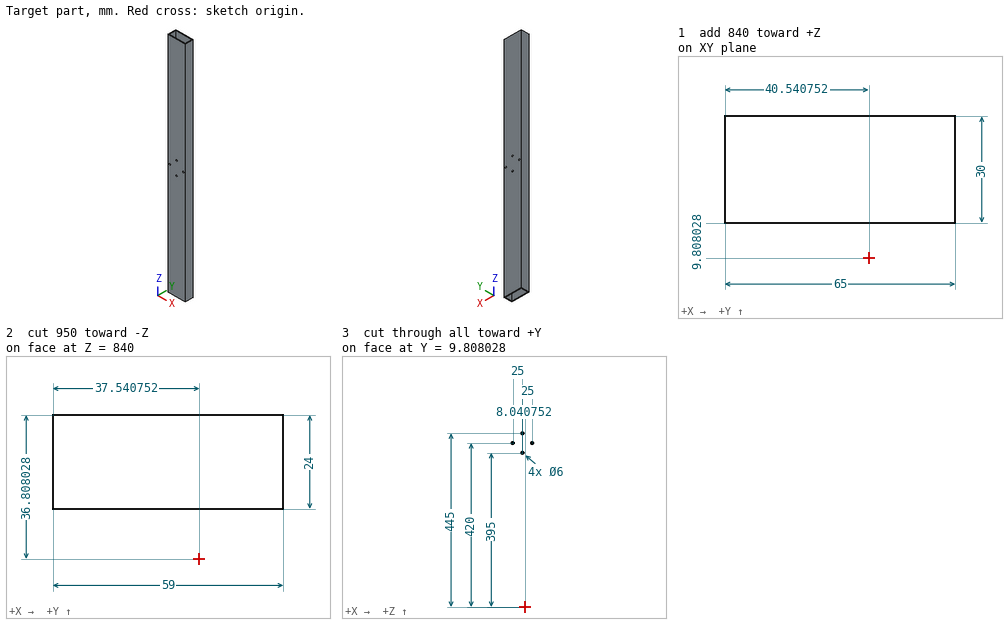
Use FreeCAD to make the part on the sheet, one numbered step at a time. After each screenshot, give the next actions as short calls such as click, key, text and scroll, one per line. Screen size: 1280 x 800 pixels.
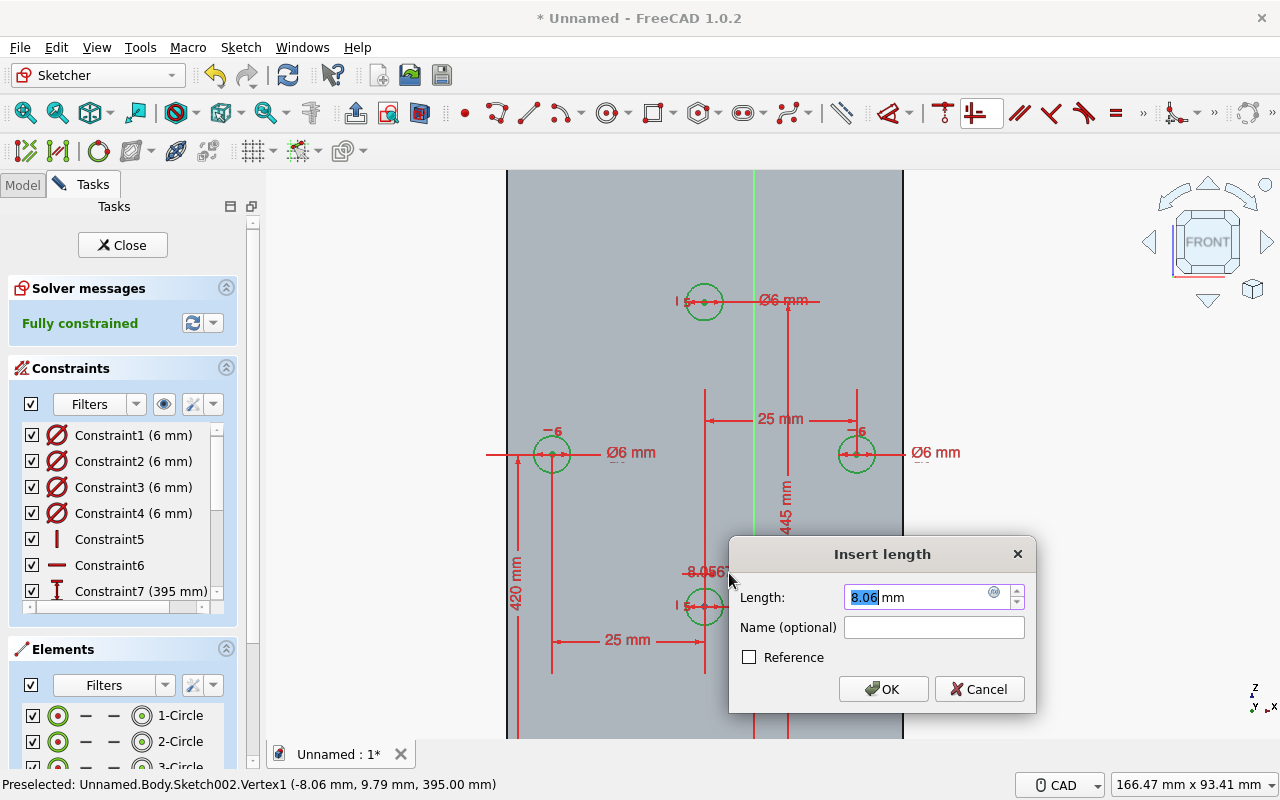
text(8.040752)
key(Return)
key(Escape)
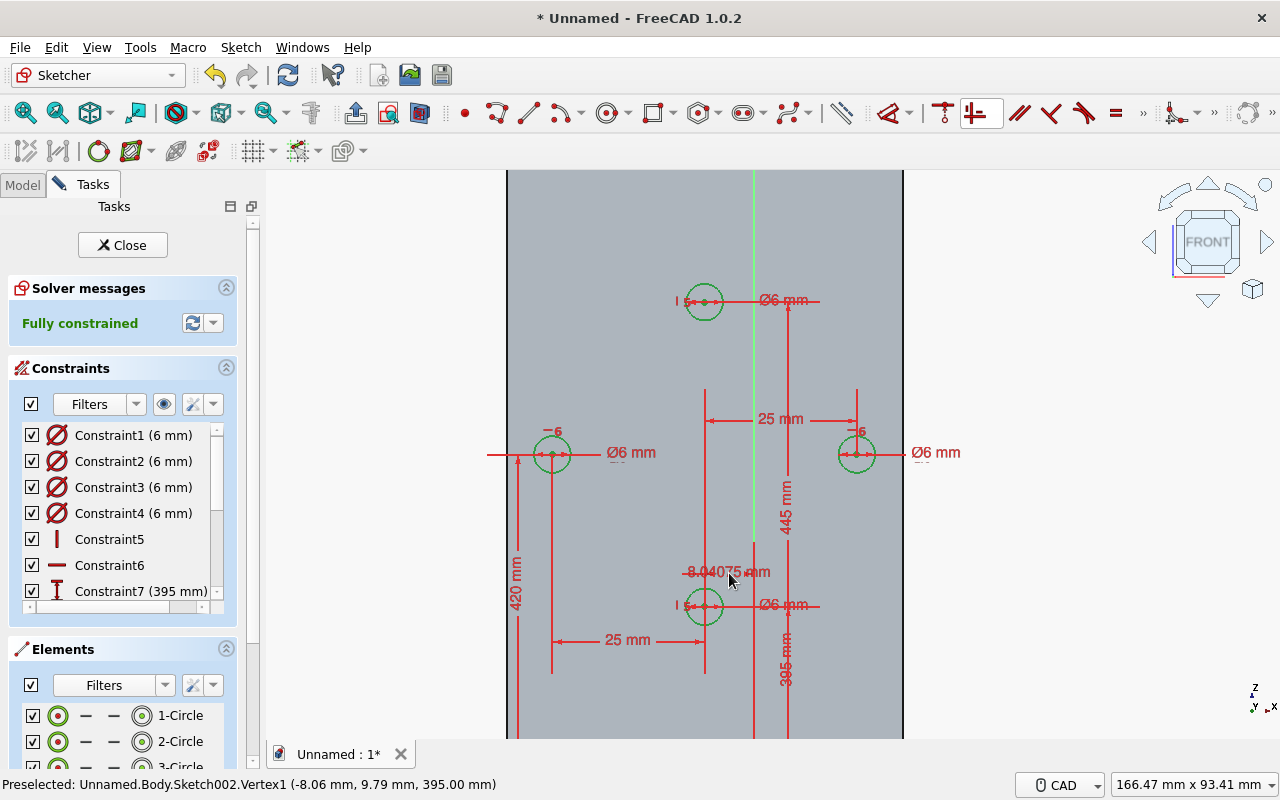
click(123, 245)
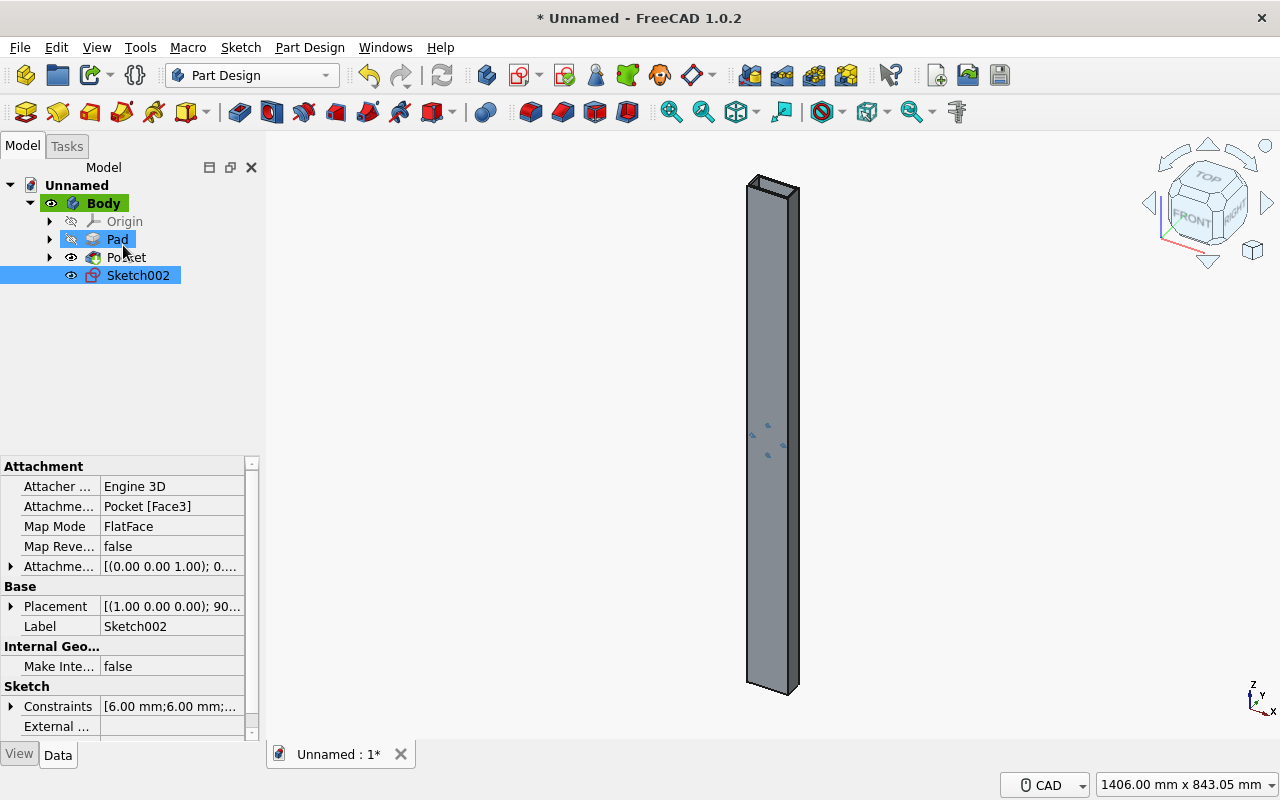
click(240, 112)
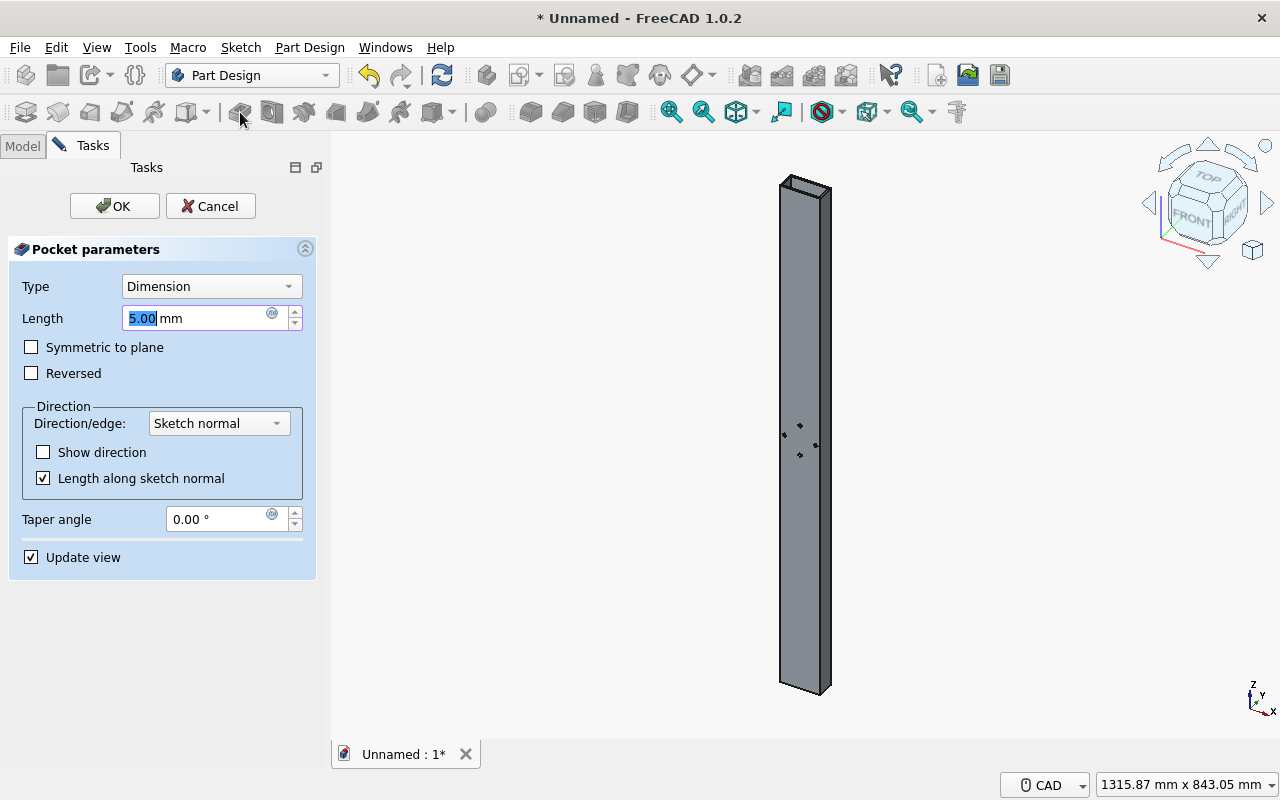
click(212, 286)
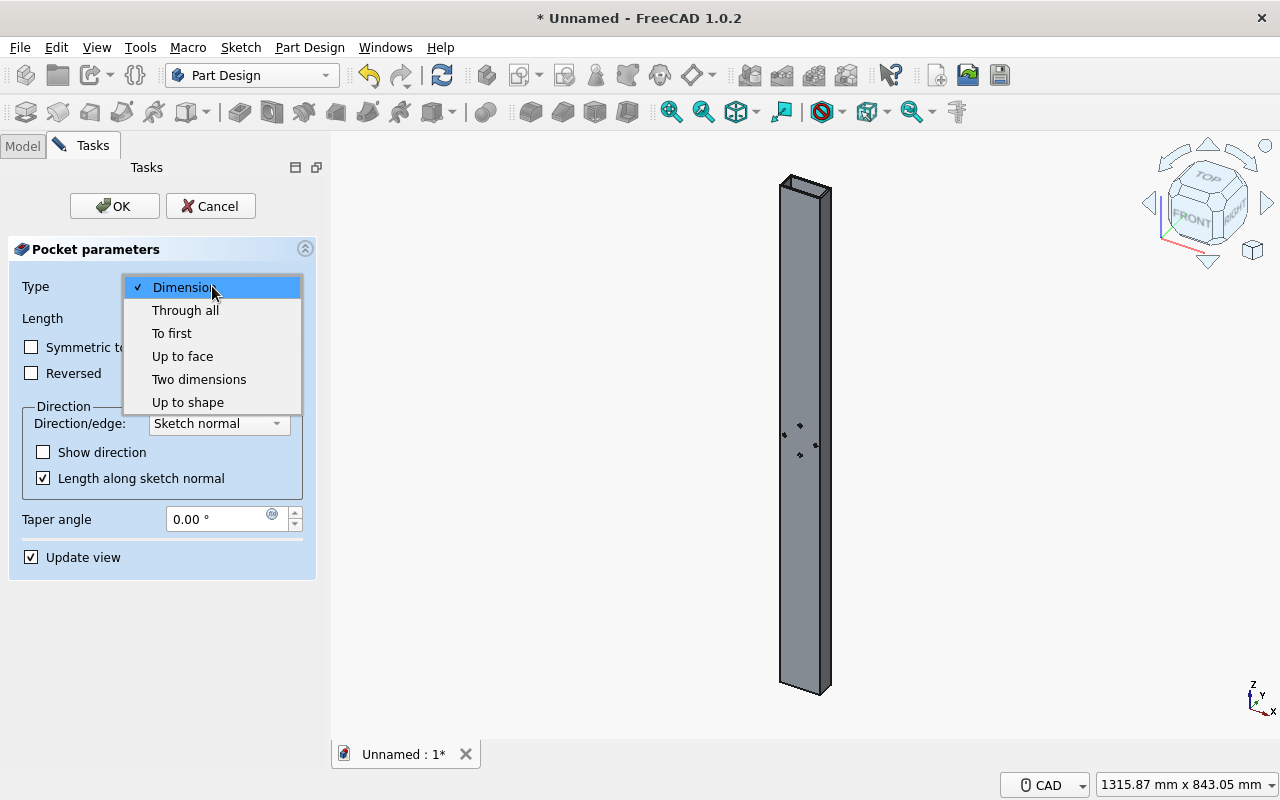
click(212, 310)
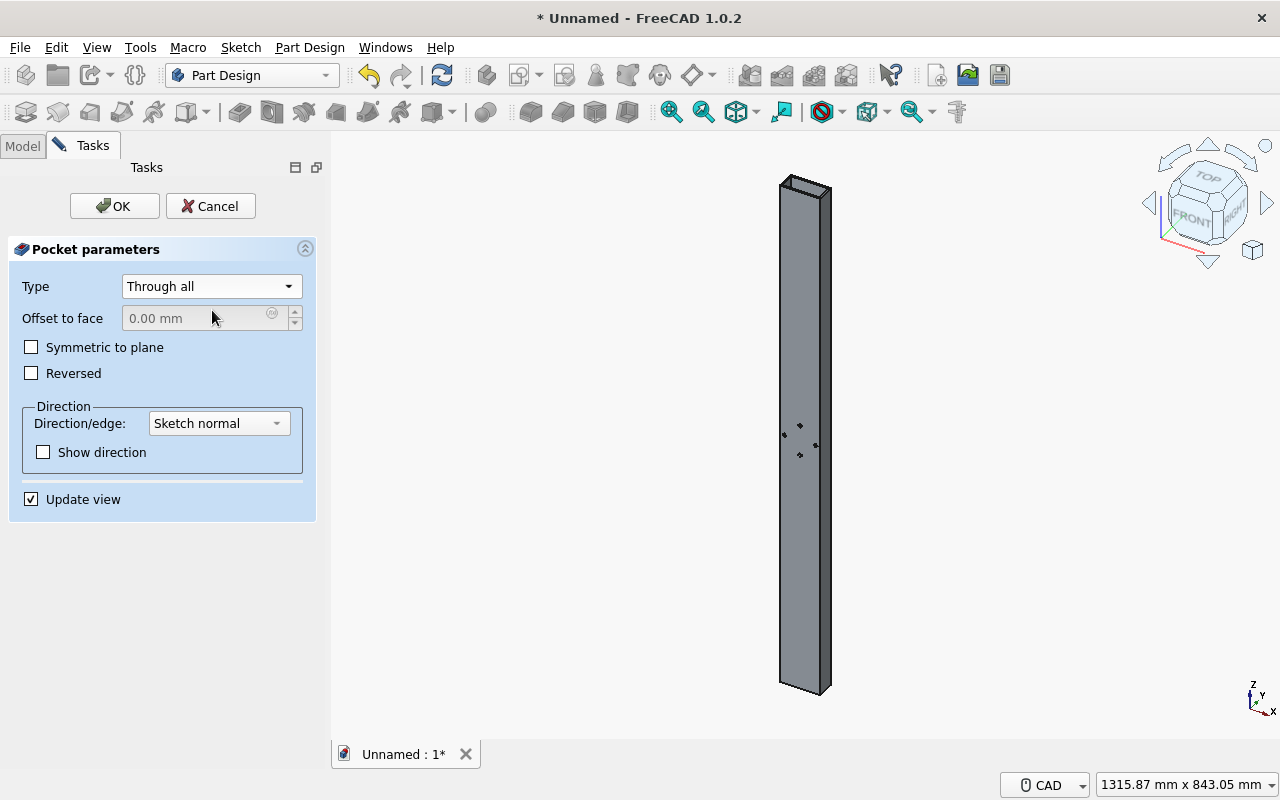
click(115, 206)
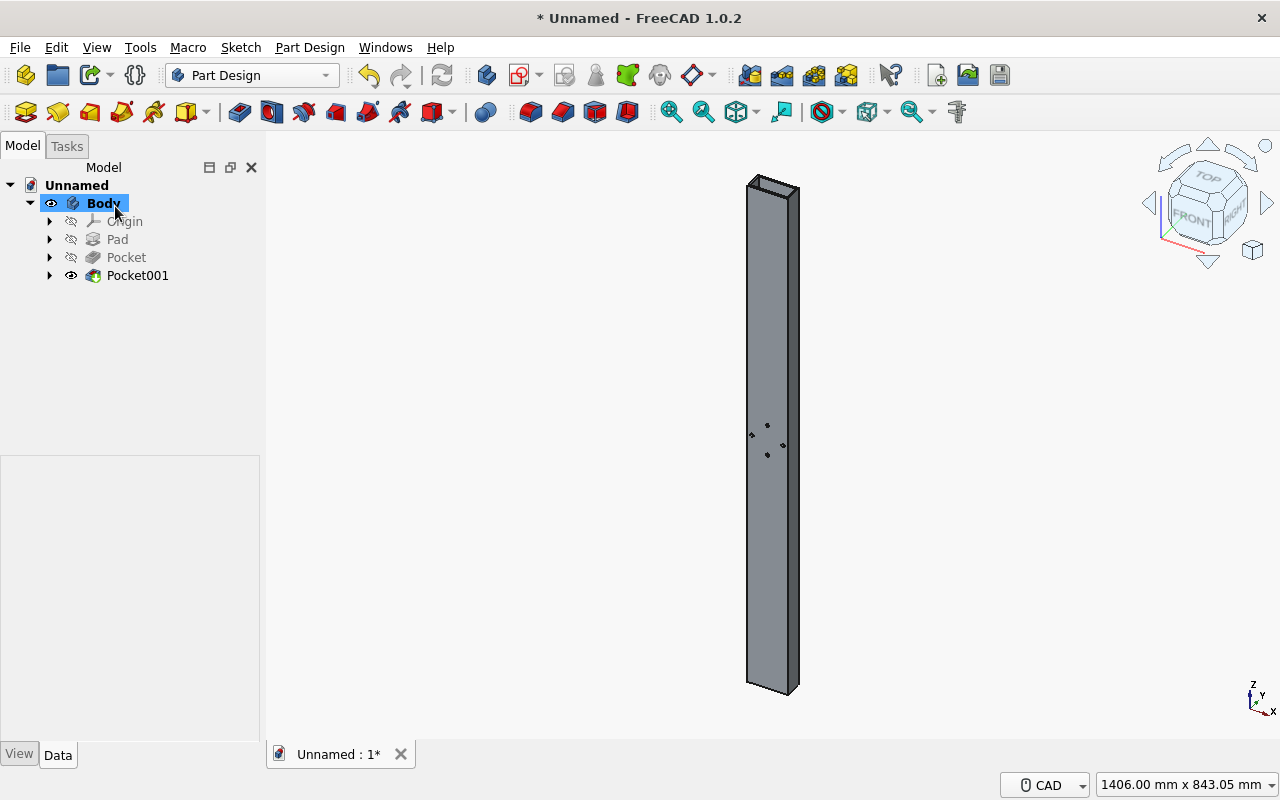
key(0)